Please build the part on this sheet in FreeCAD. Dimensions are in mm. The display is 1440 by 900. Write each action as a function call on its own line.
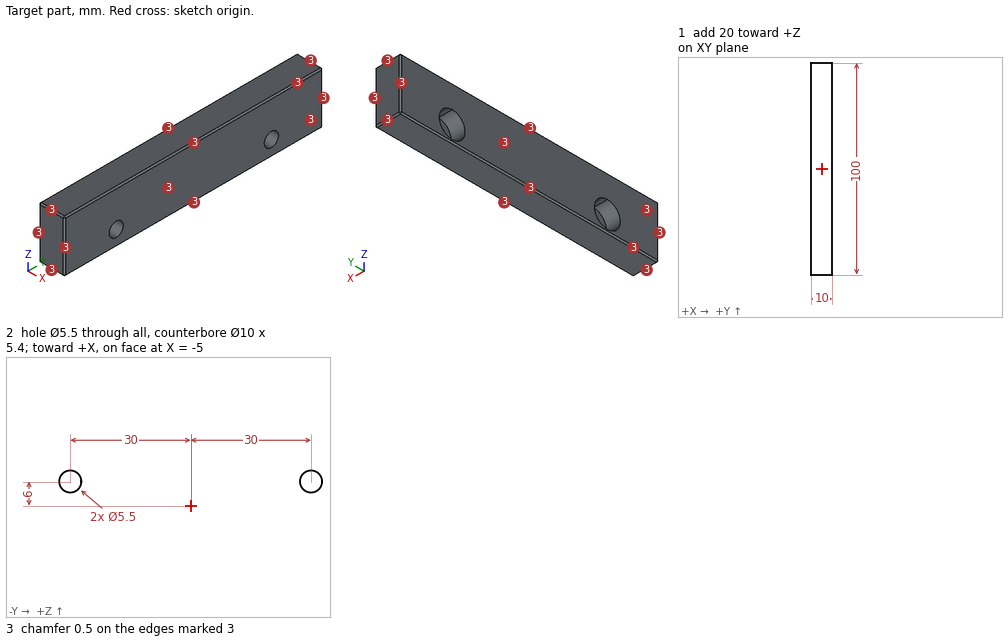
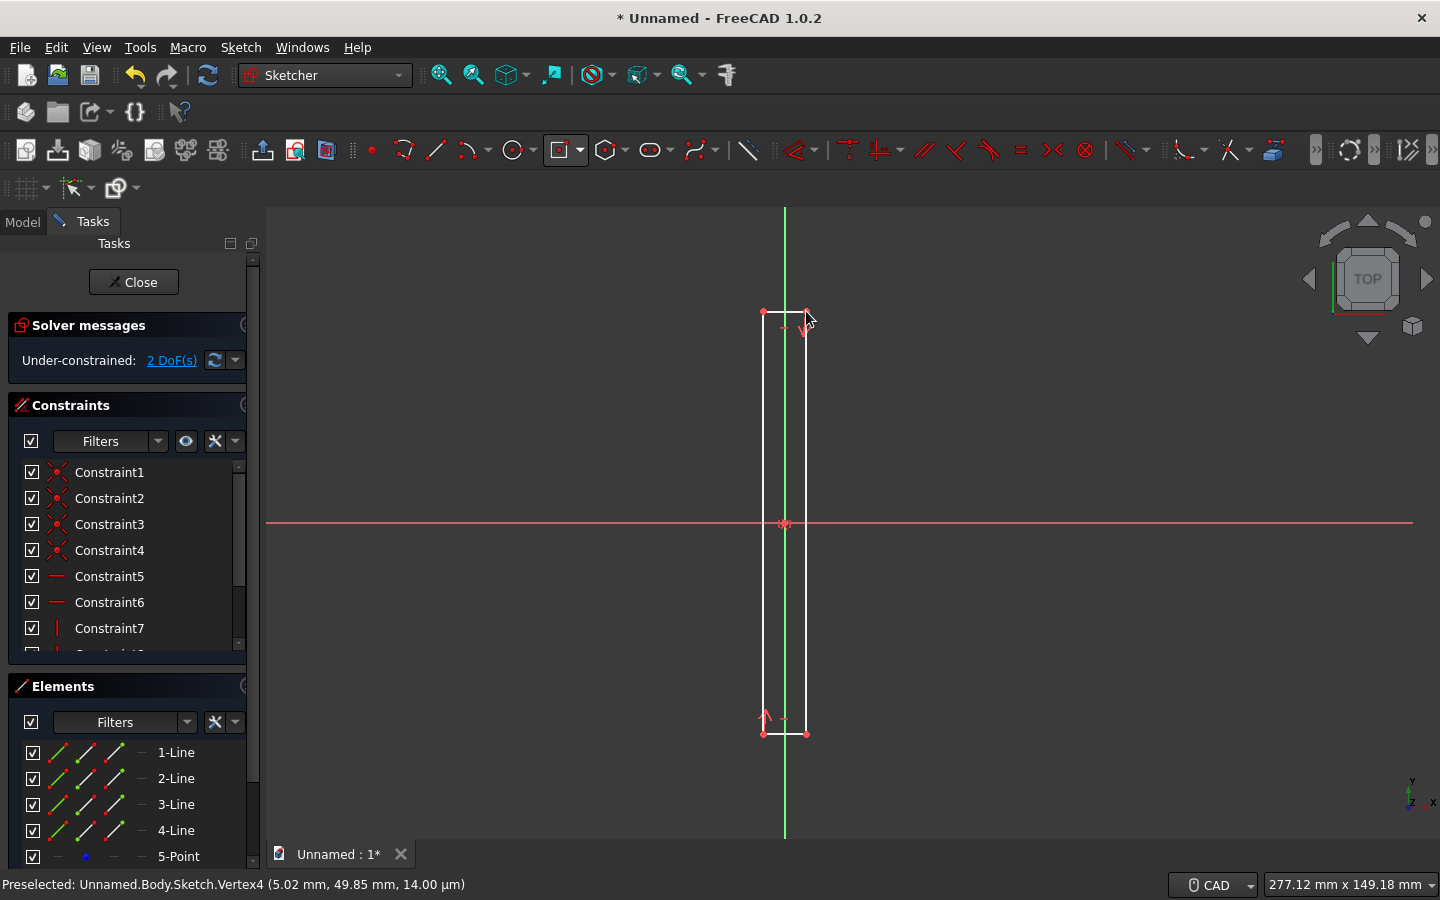
click(794, 150)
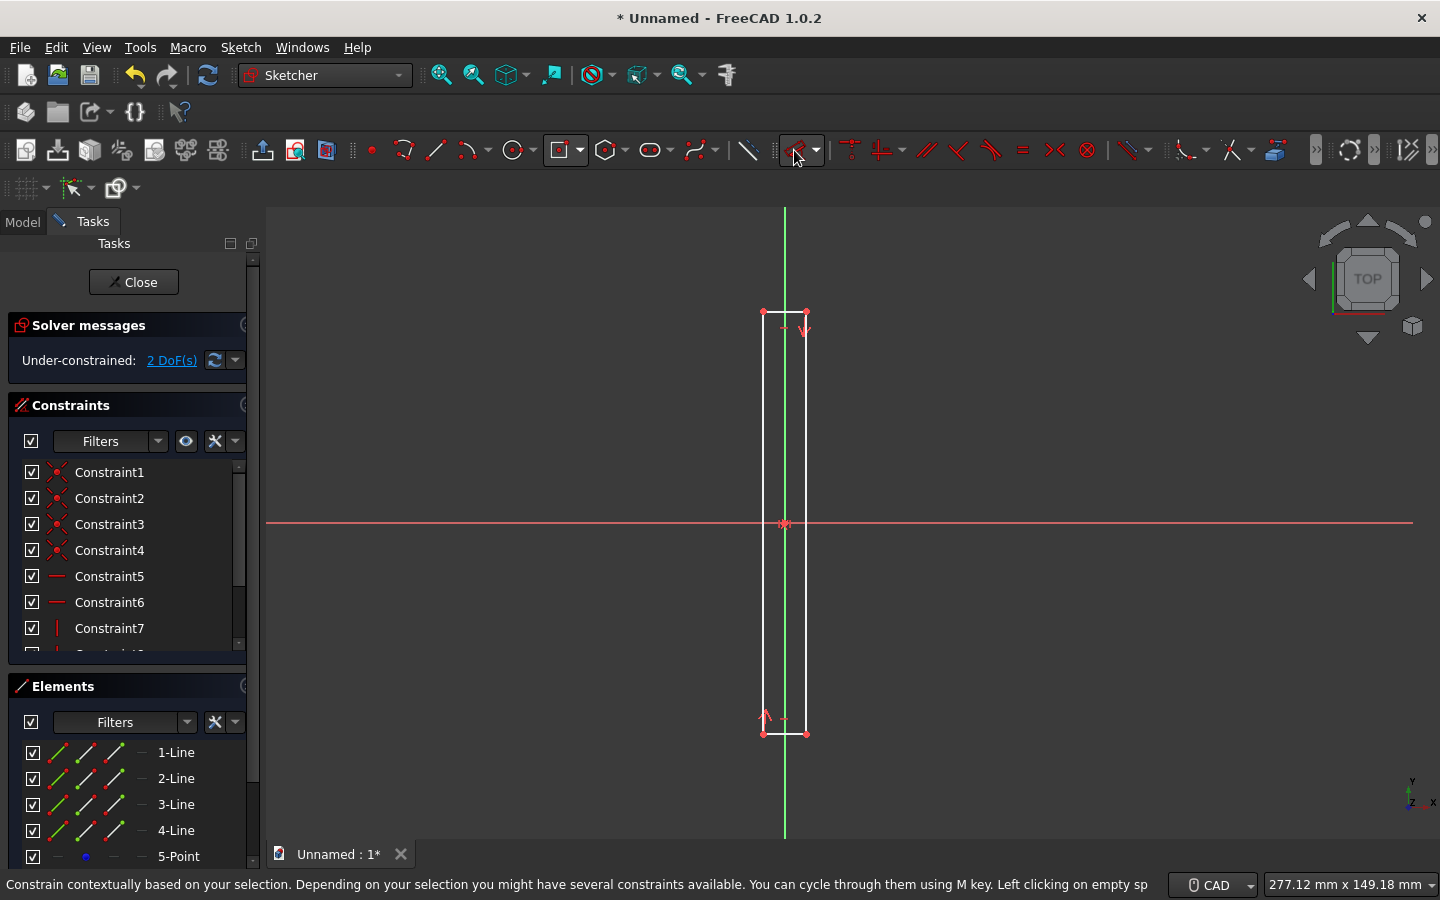
click(785, 734)
click(770, 768)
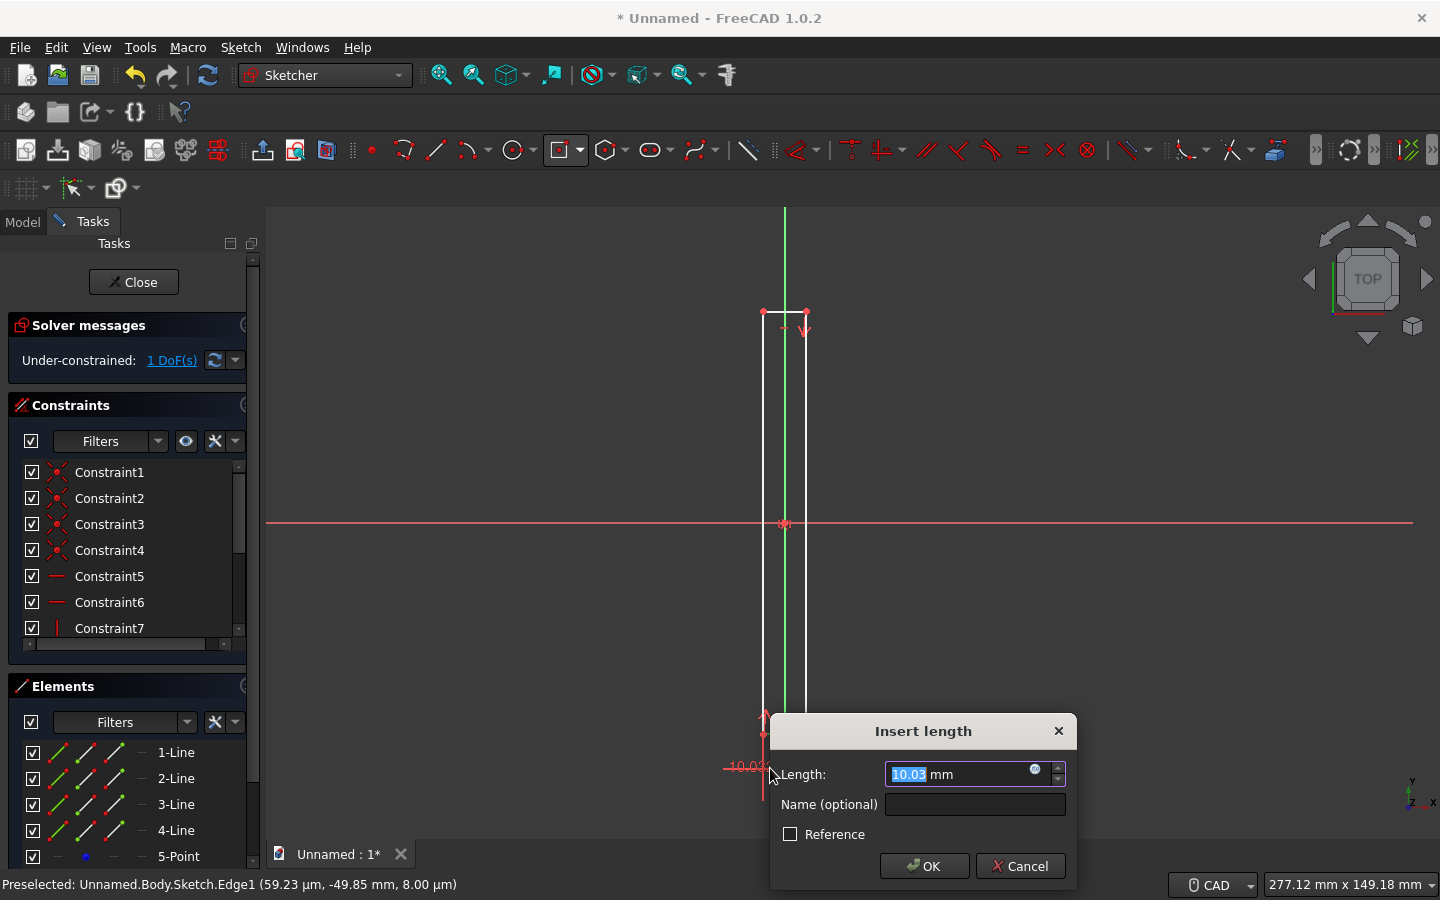
text(10)
key(Return)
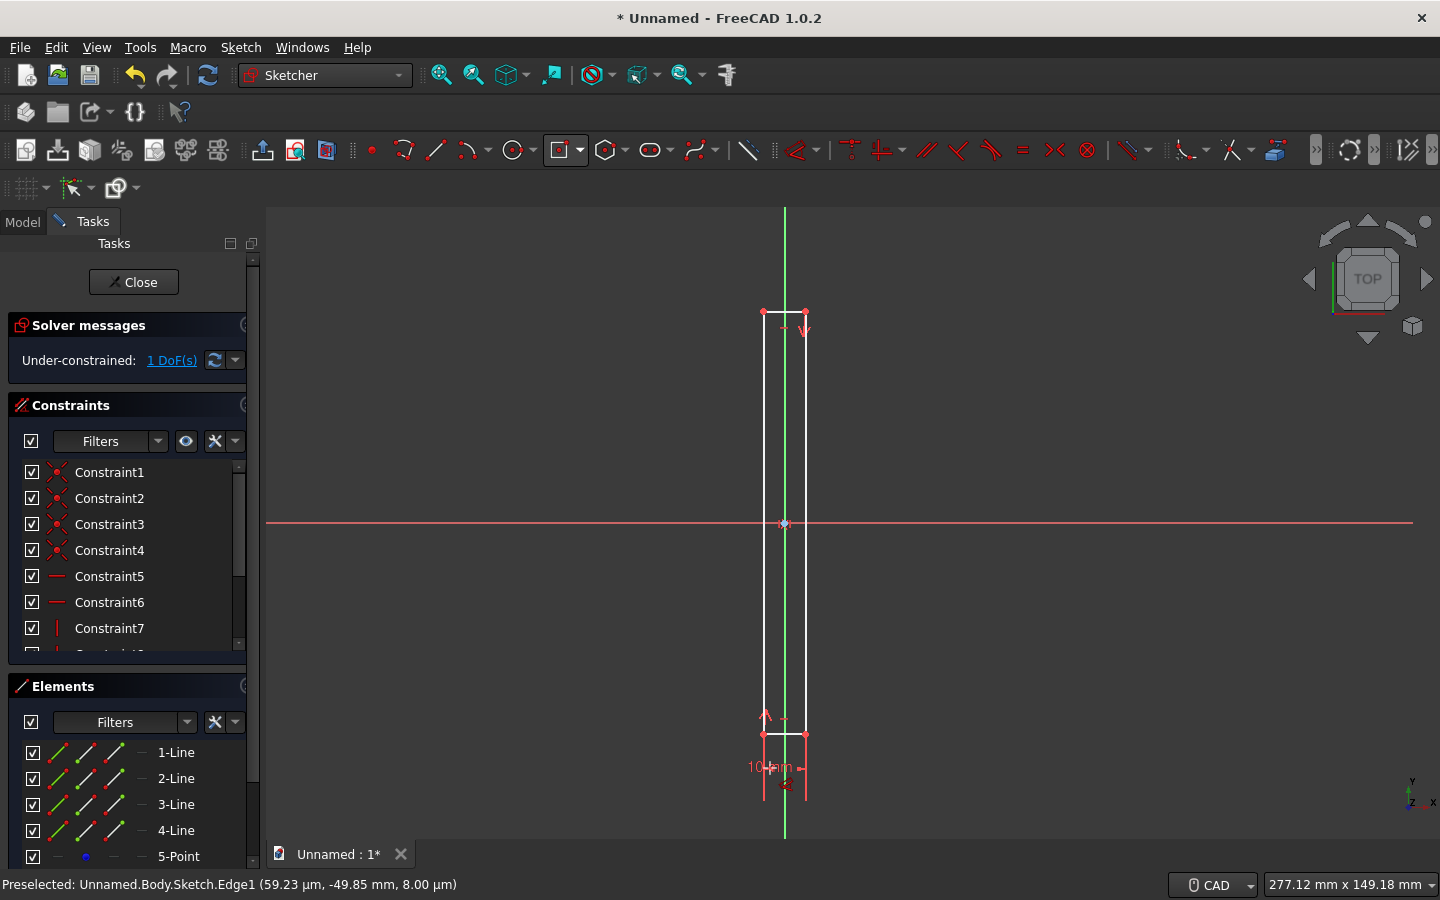
click(806, 608)
click(840, 426)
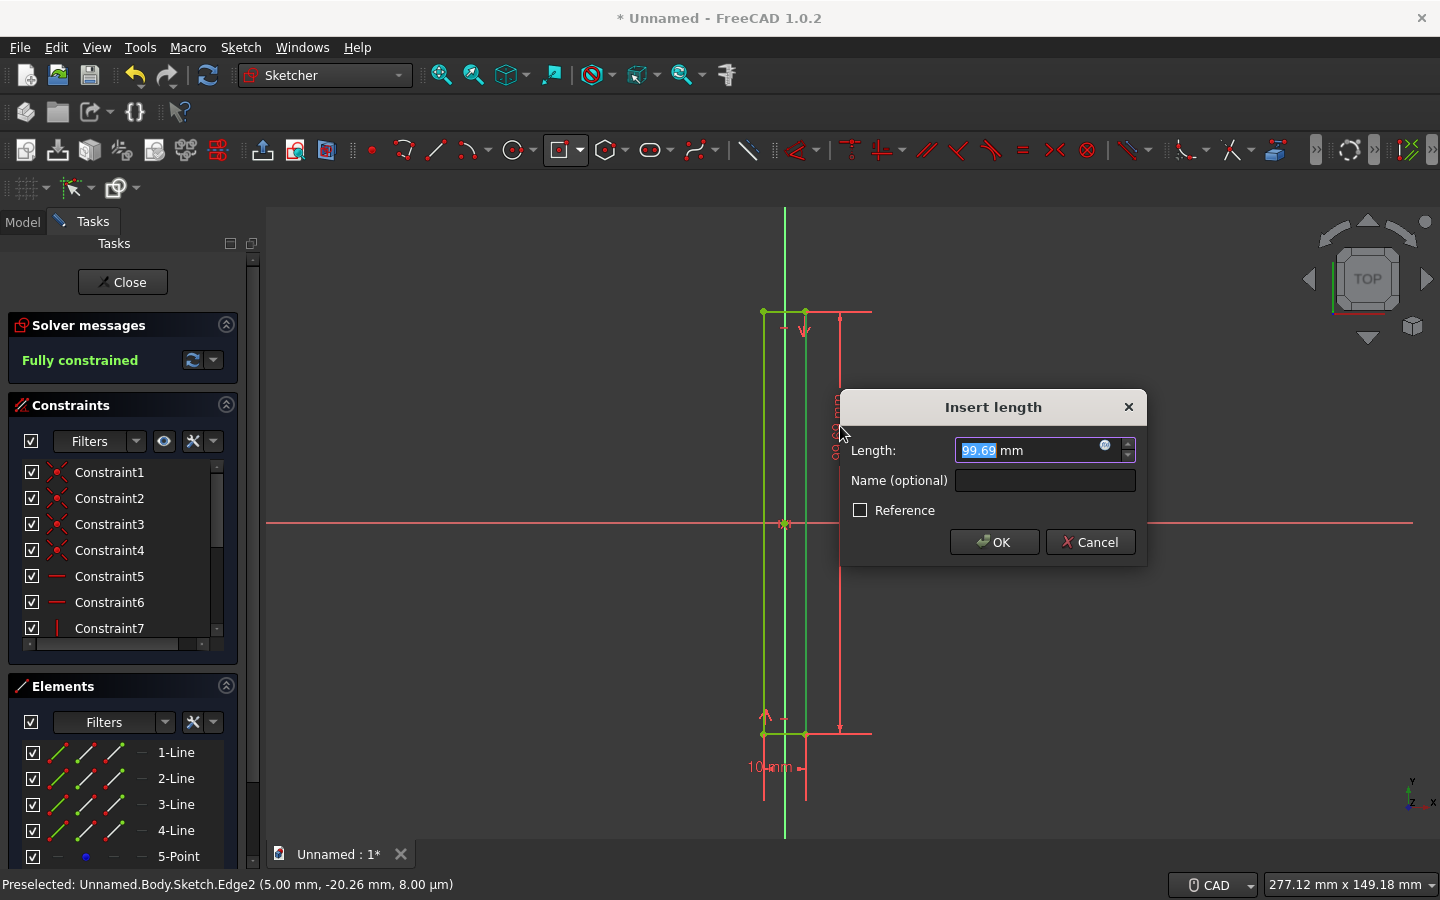
text(100)
key(Return)
key(Escape)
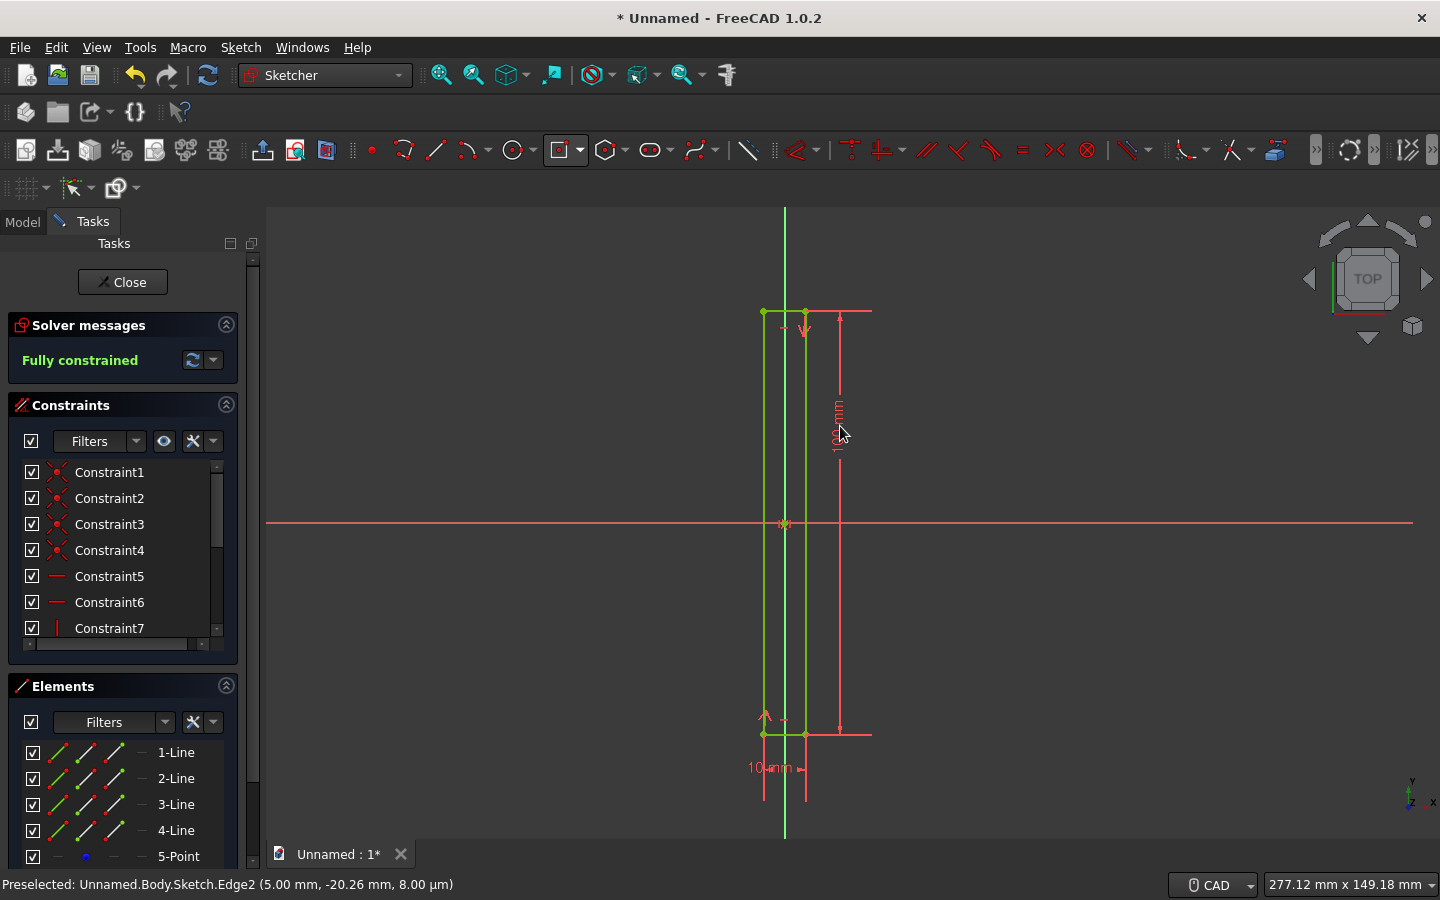
click(123, 282)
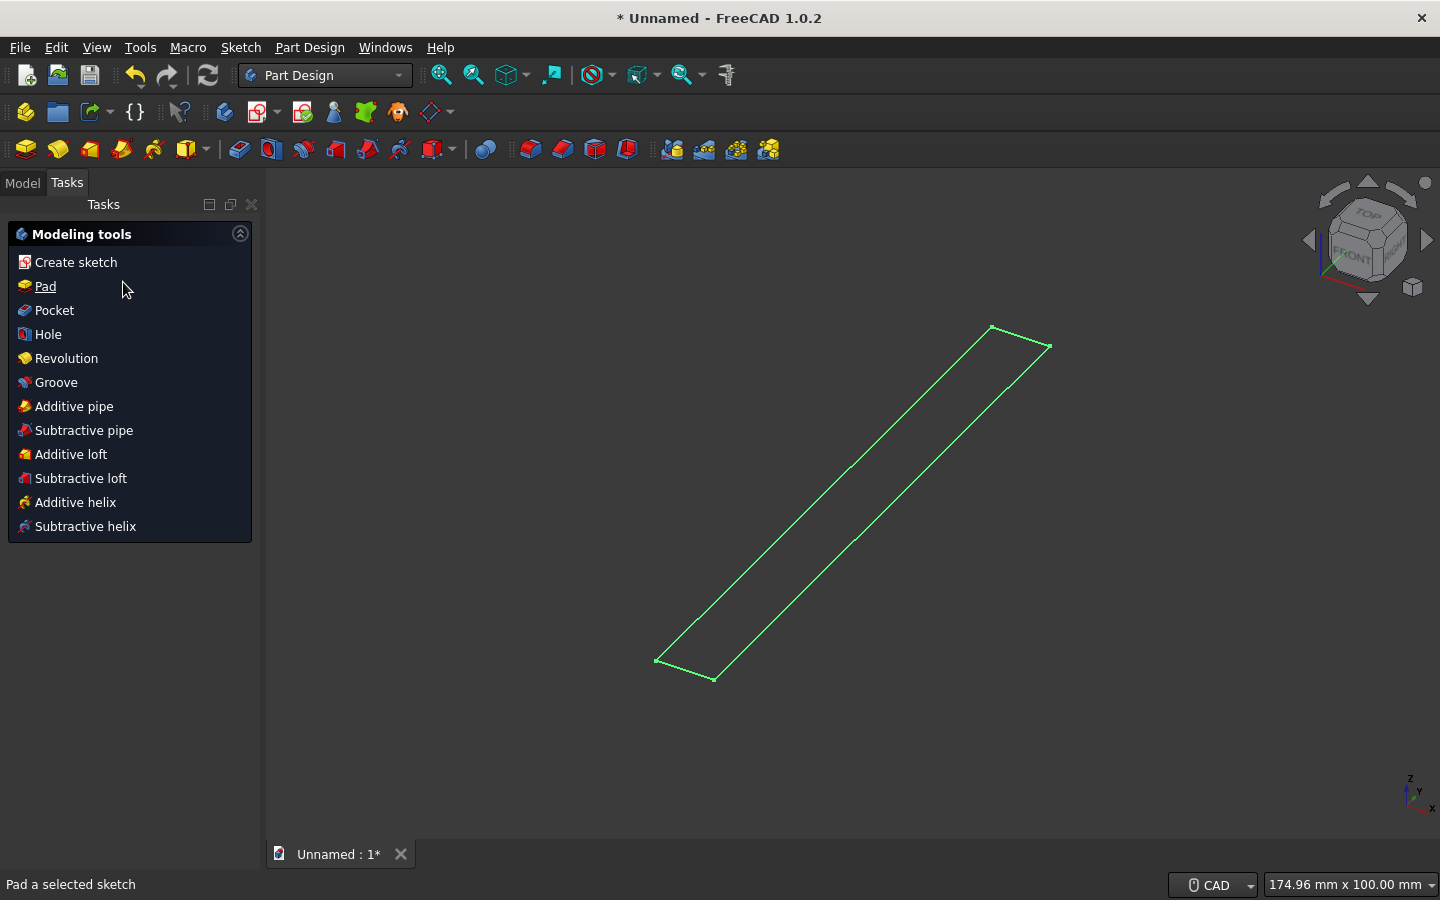
click(26, 150)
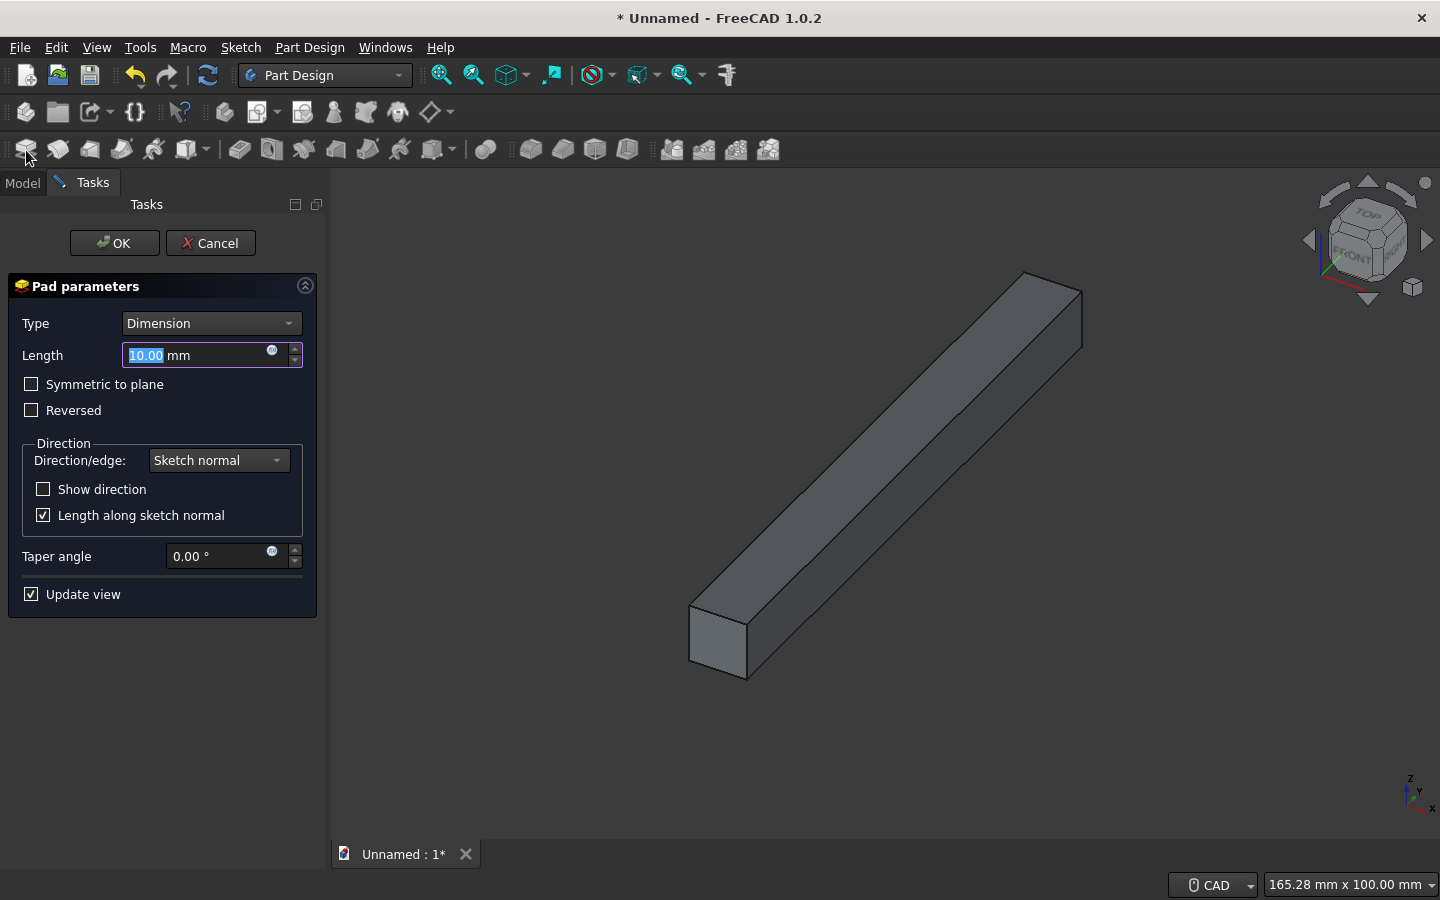
text(20)
key(Tab)